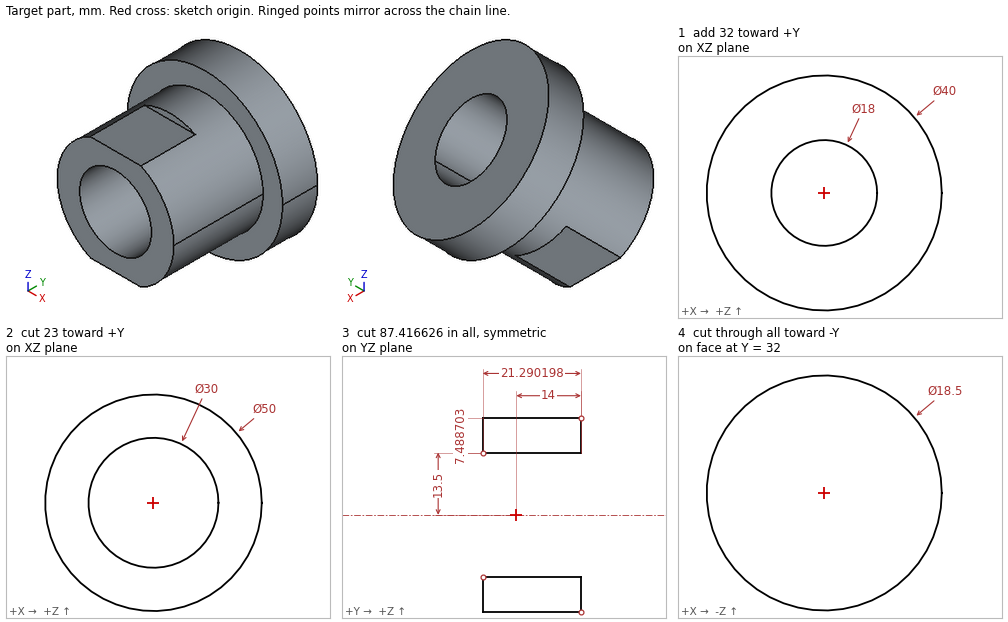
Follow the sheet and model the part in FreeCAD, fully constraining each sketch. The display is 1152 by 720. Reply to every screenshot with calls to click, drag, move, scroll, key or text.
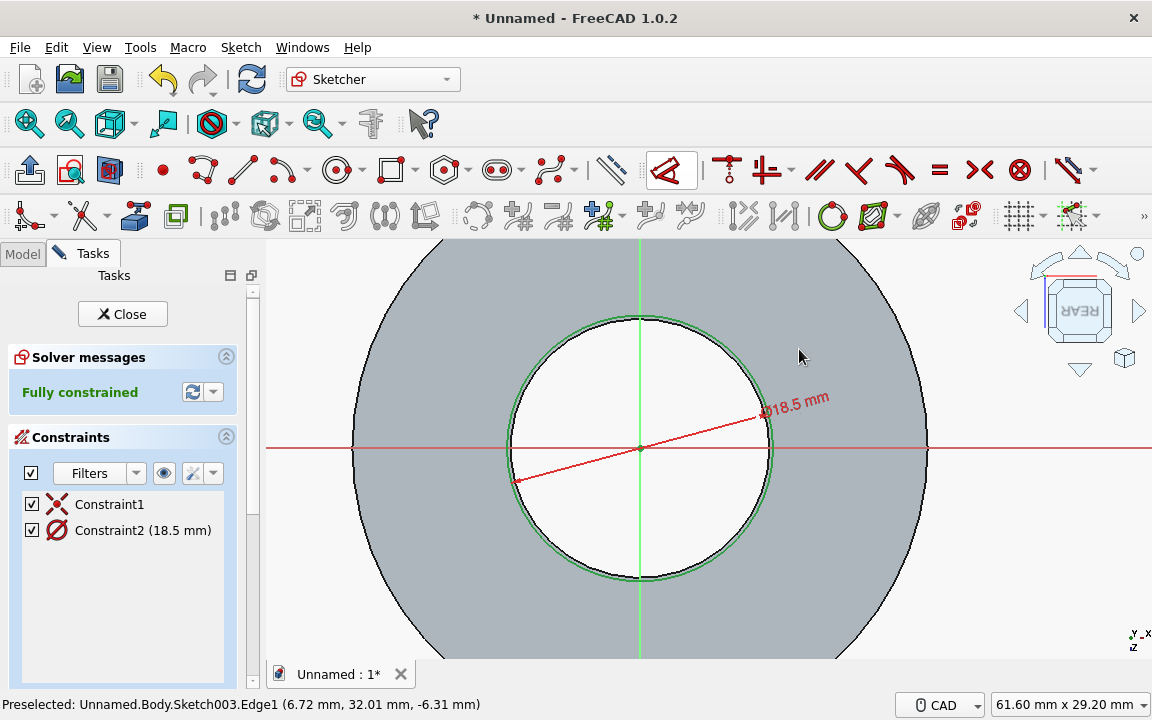
click(123, 314)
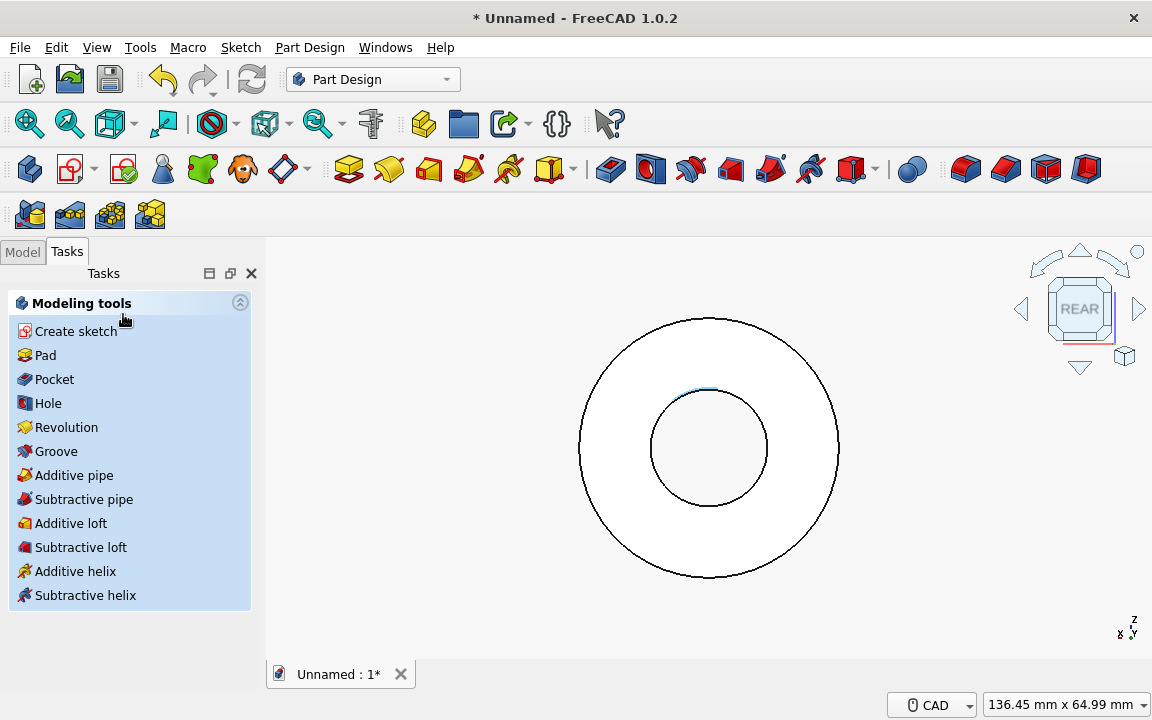
click(612, 170)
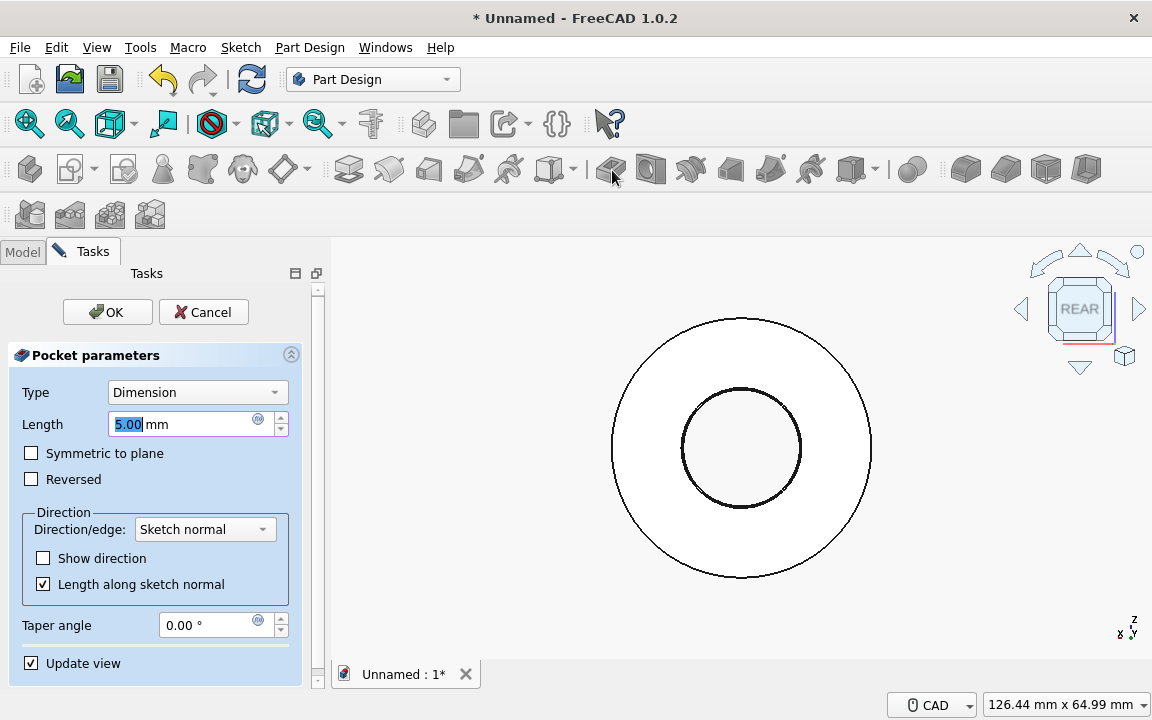
click(198, 392)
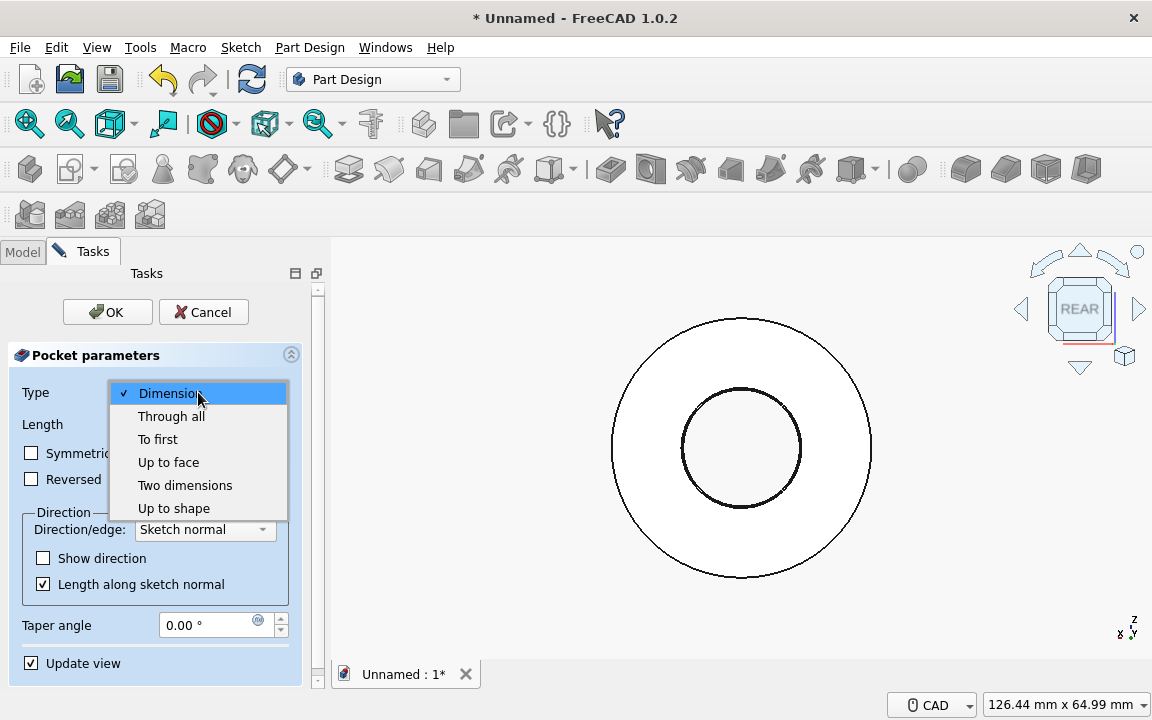
click(198, 416)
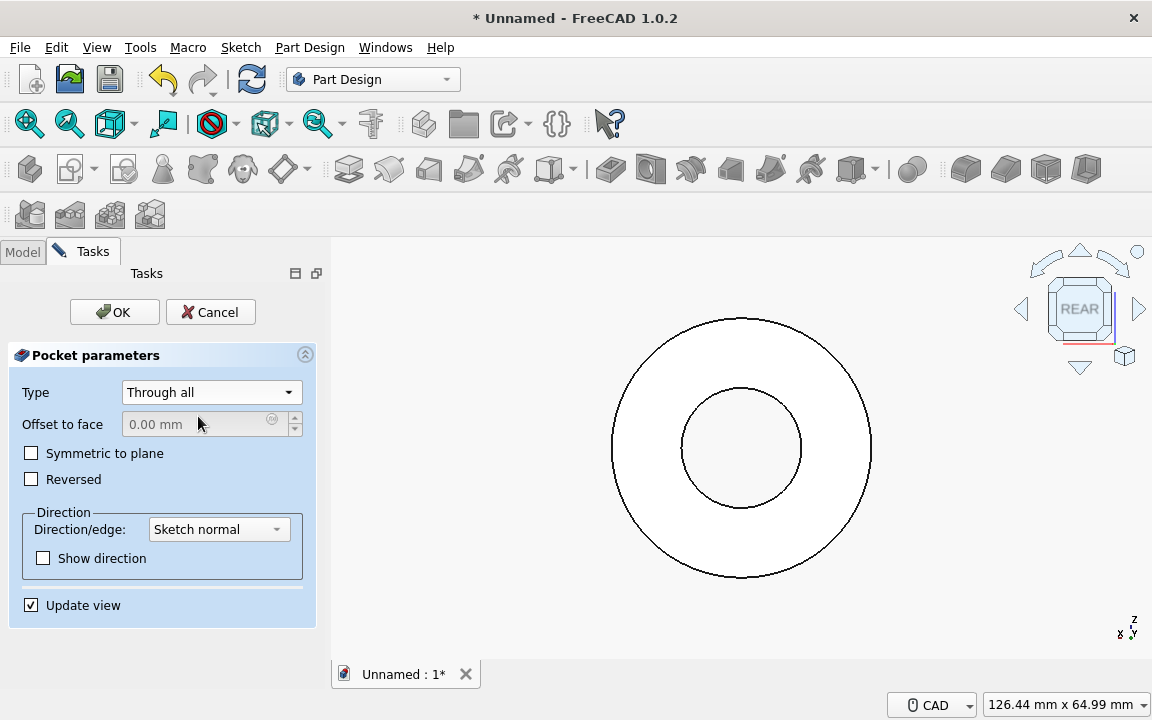
click(115, 312)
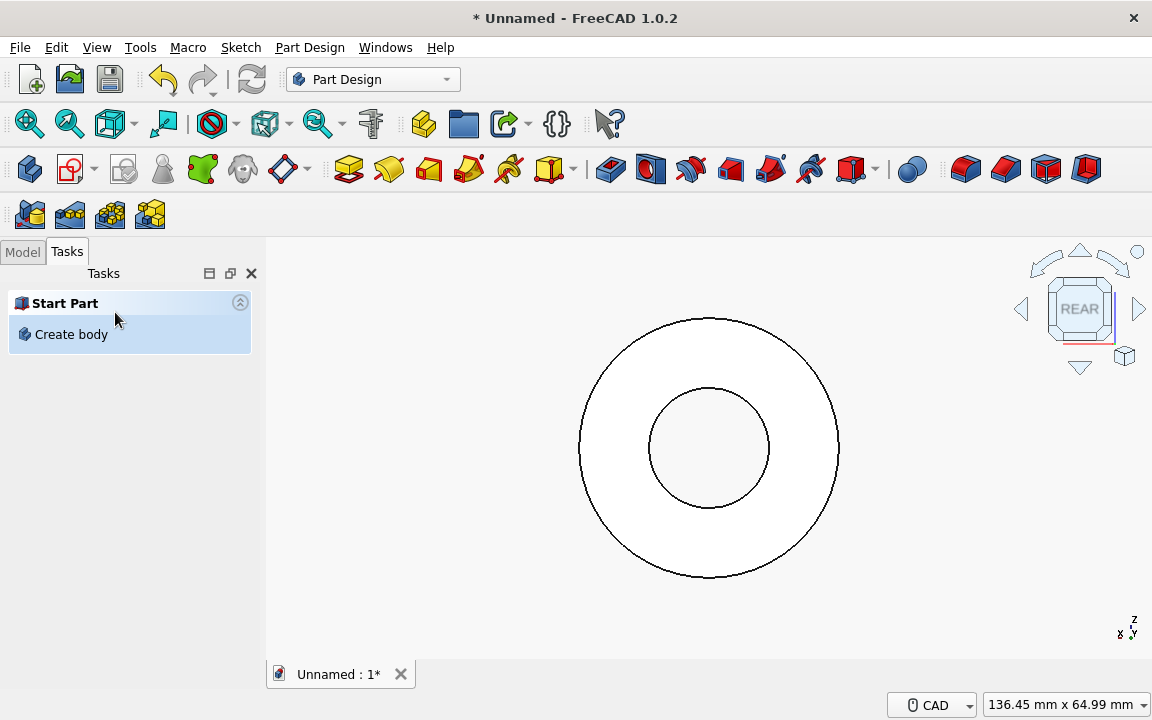
key(0)